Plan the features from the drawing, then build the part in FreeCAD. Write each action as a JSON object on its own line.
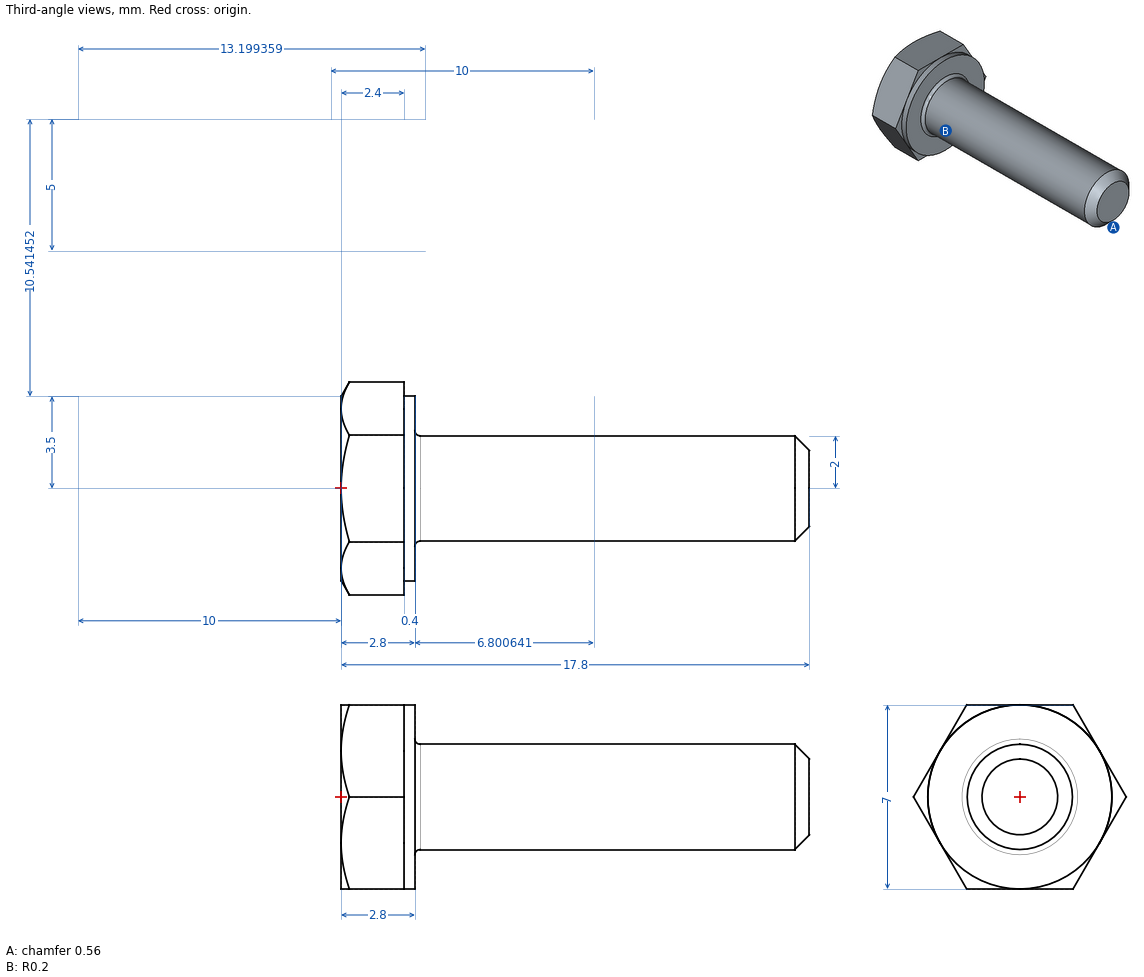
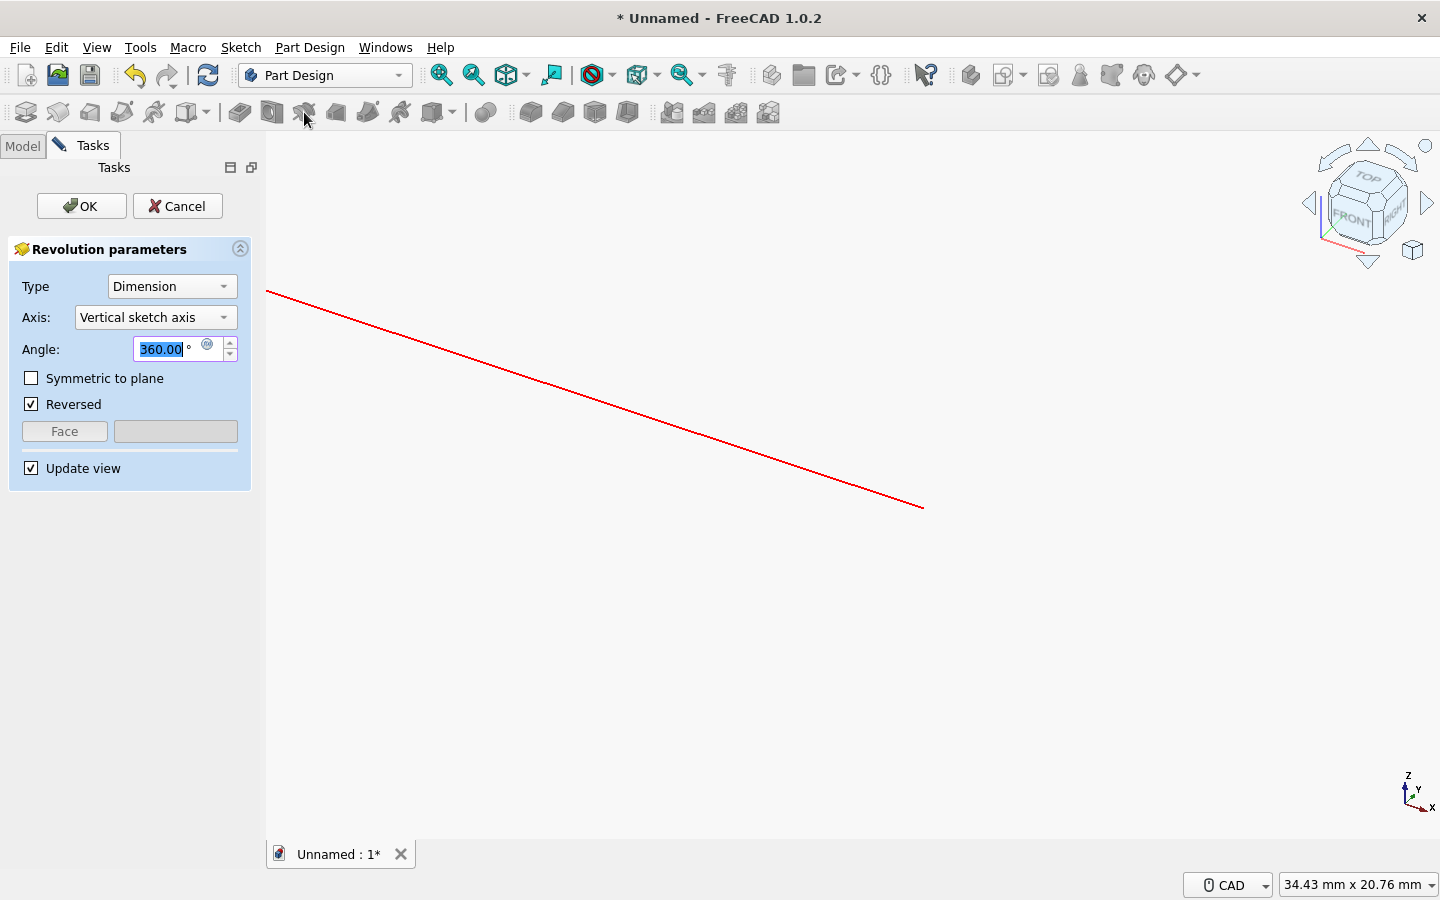
{"action": "left_click", "coordinate": [156, 318]}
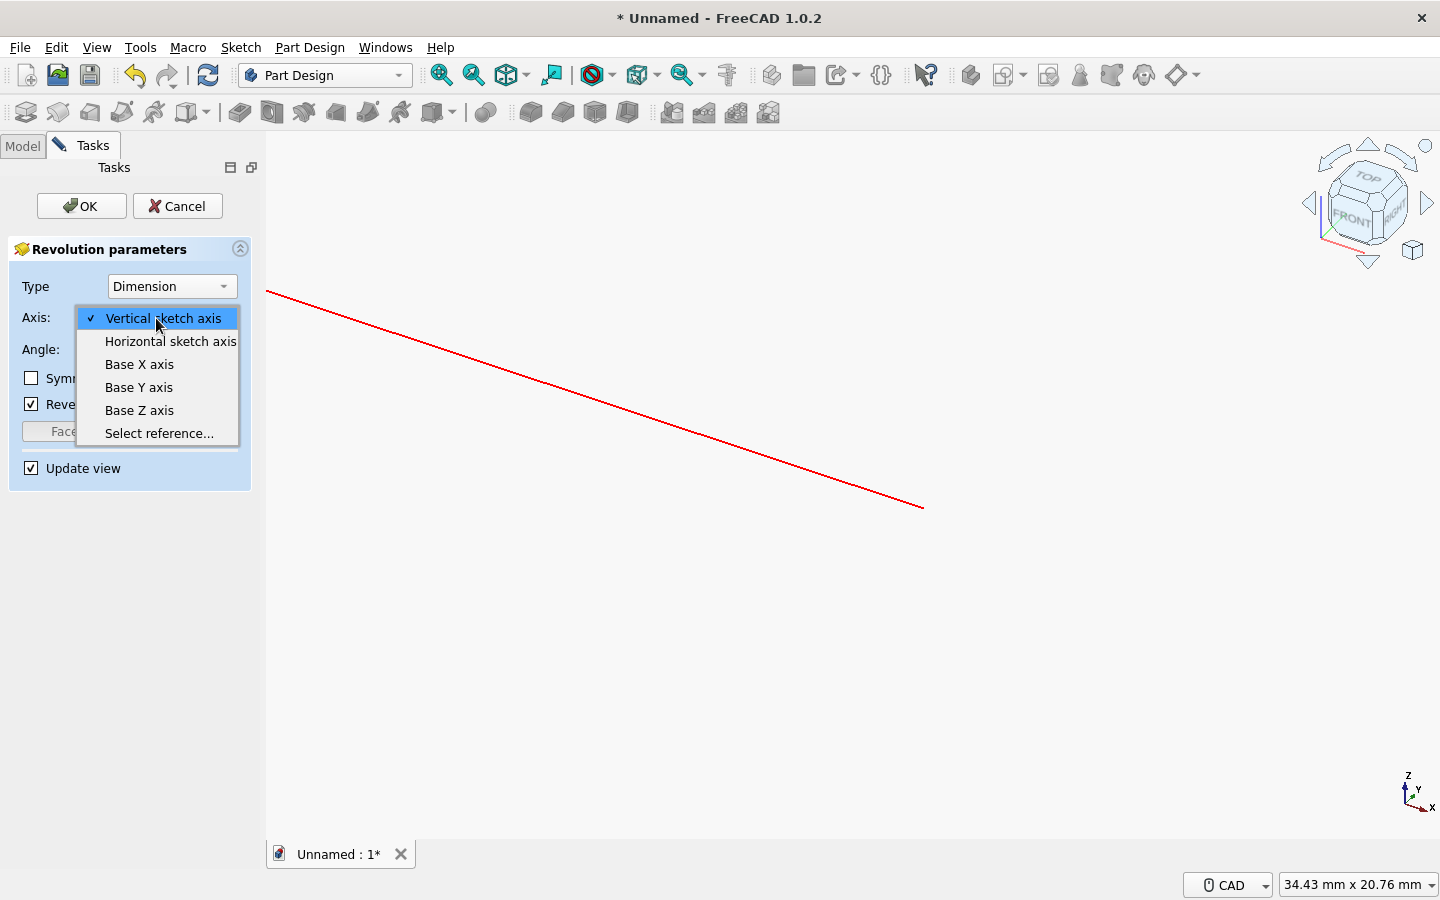
{"action": "left_click", "coordinate": [156, 342]}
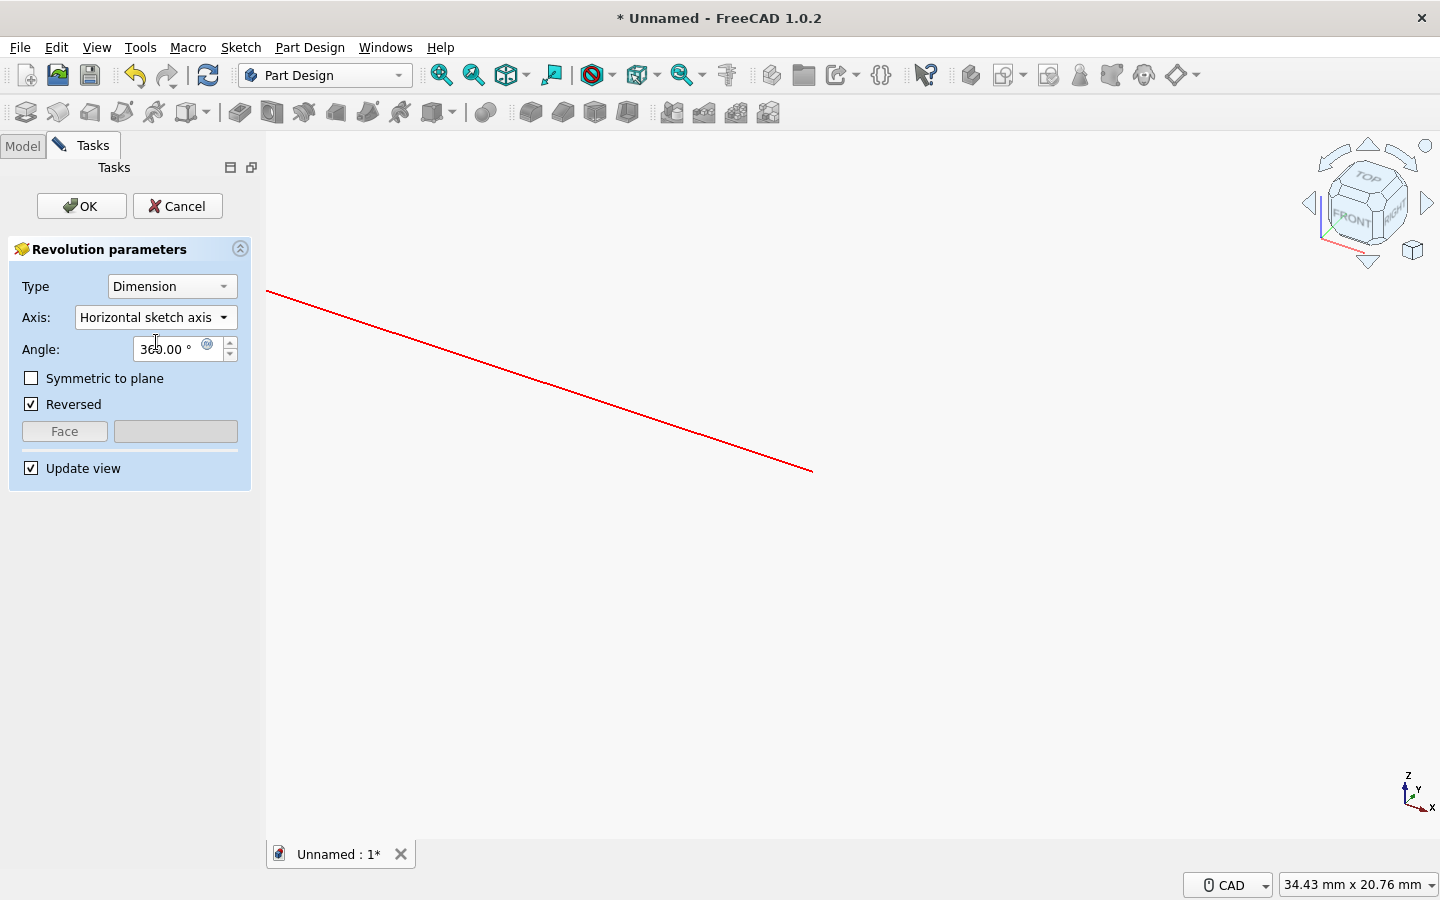
{"action": "left_click", "coordinate": [82, 206]}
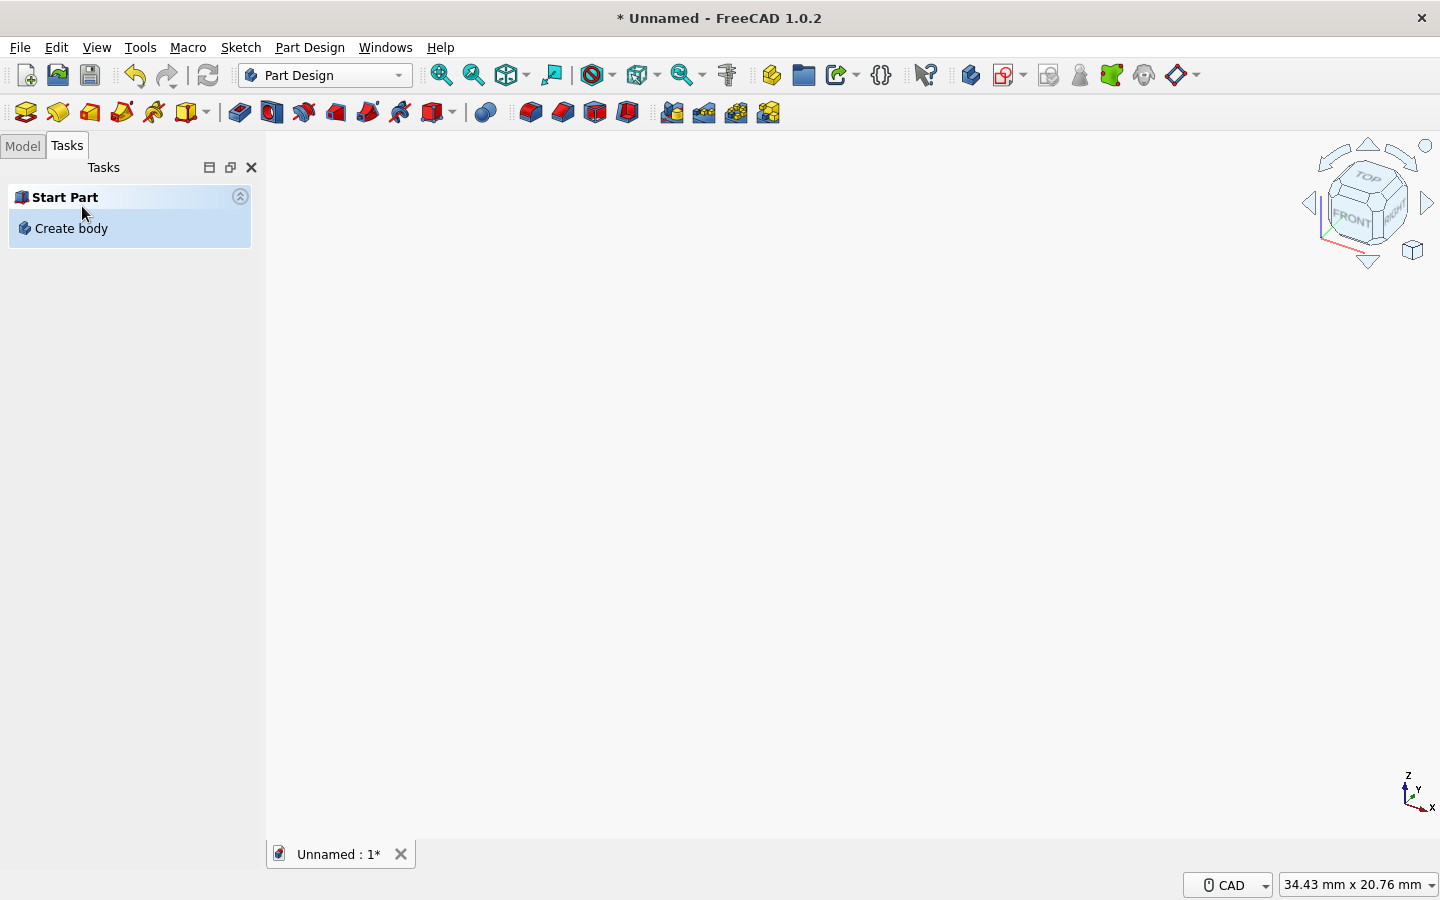
{"action": "key", "text": "v f"}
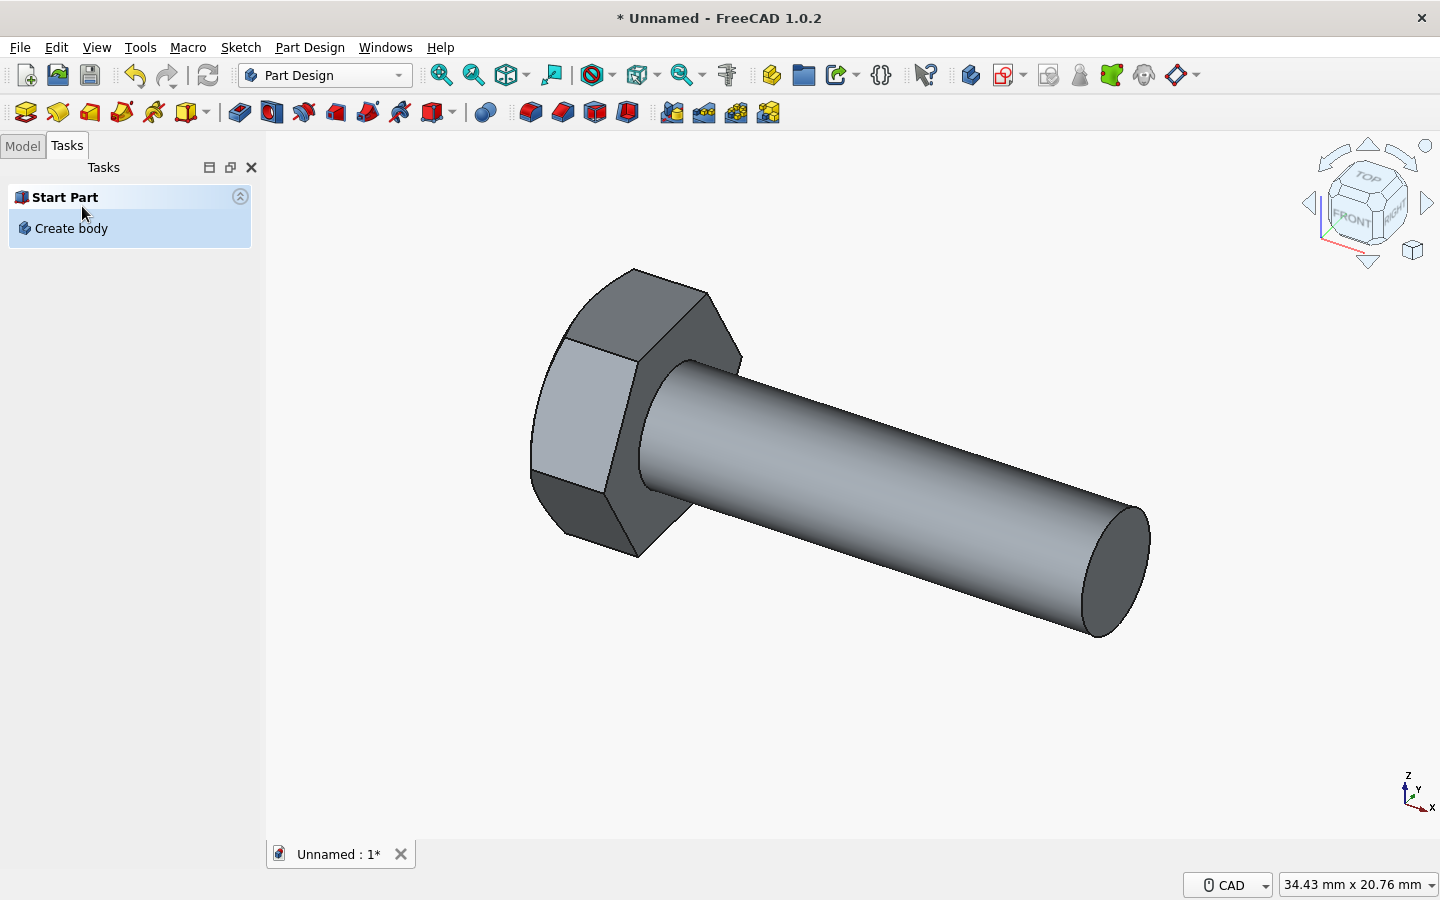
{"action": "left_click", "coordinate": [1004, 76]}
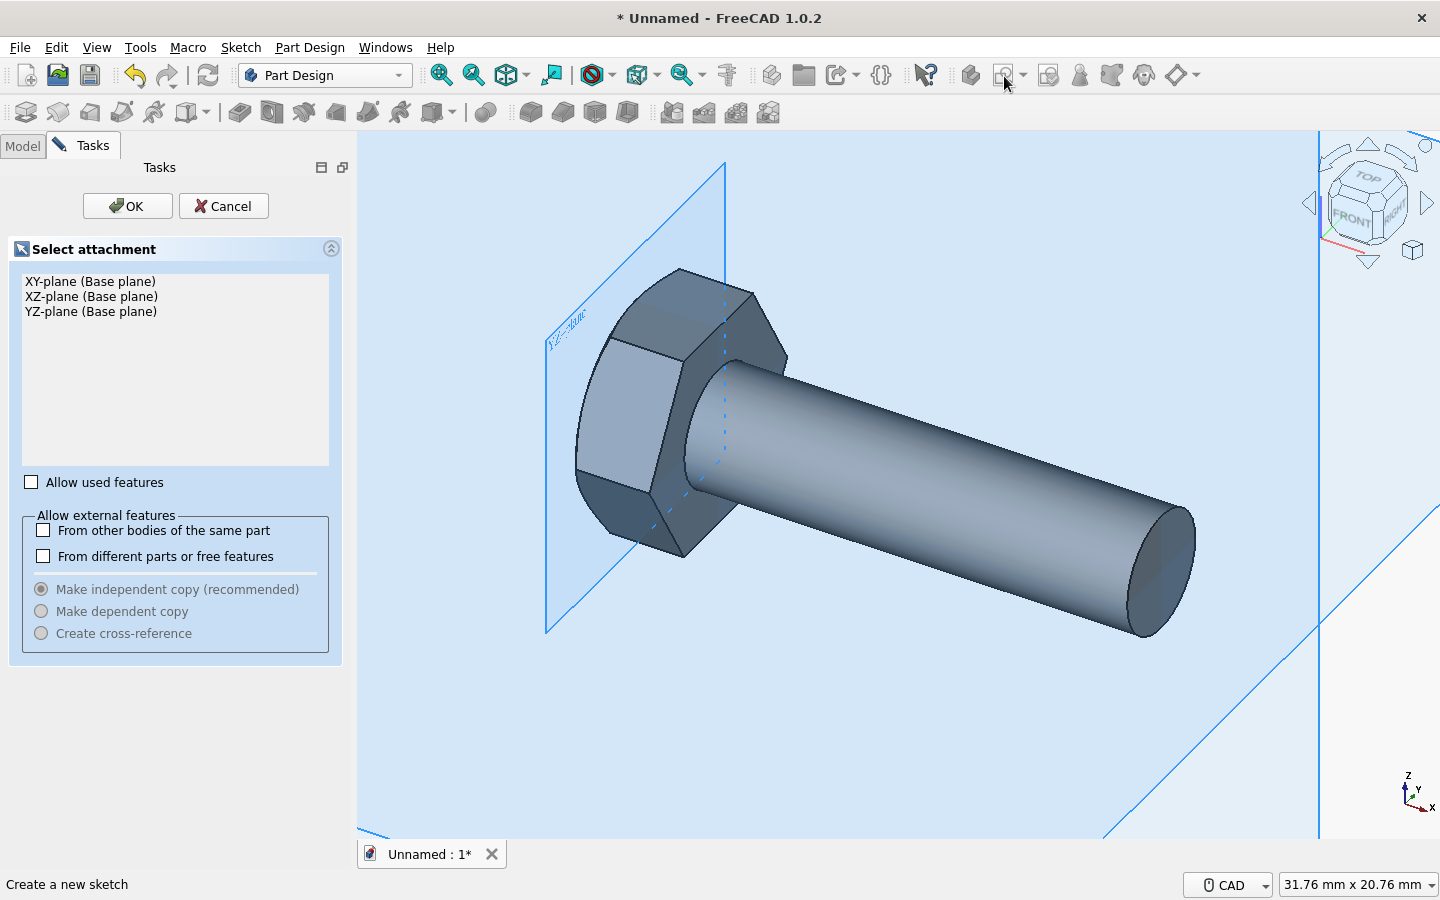
{"action": "left_click", "coordinate": [82, 282]}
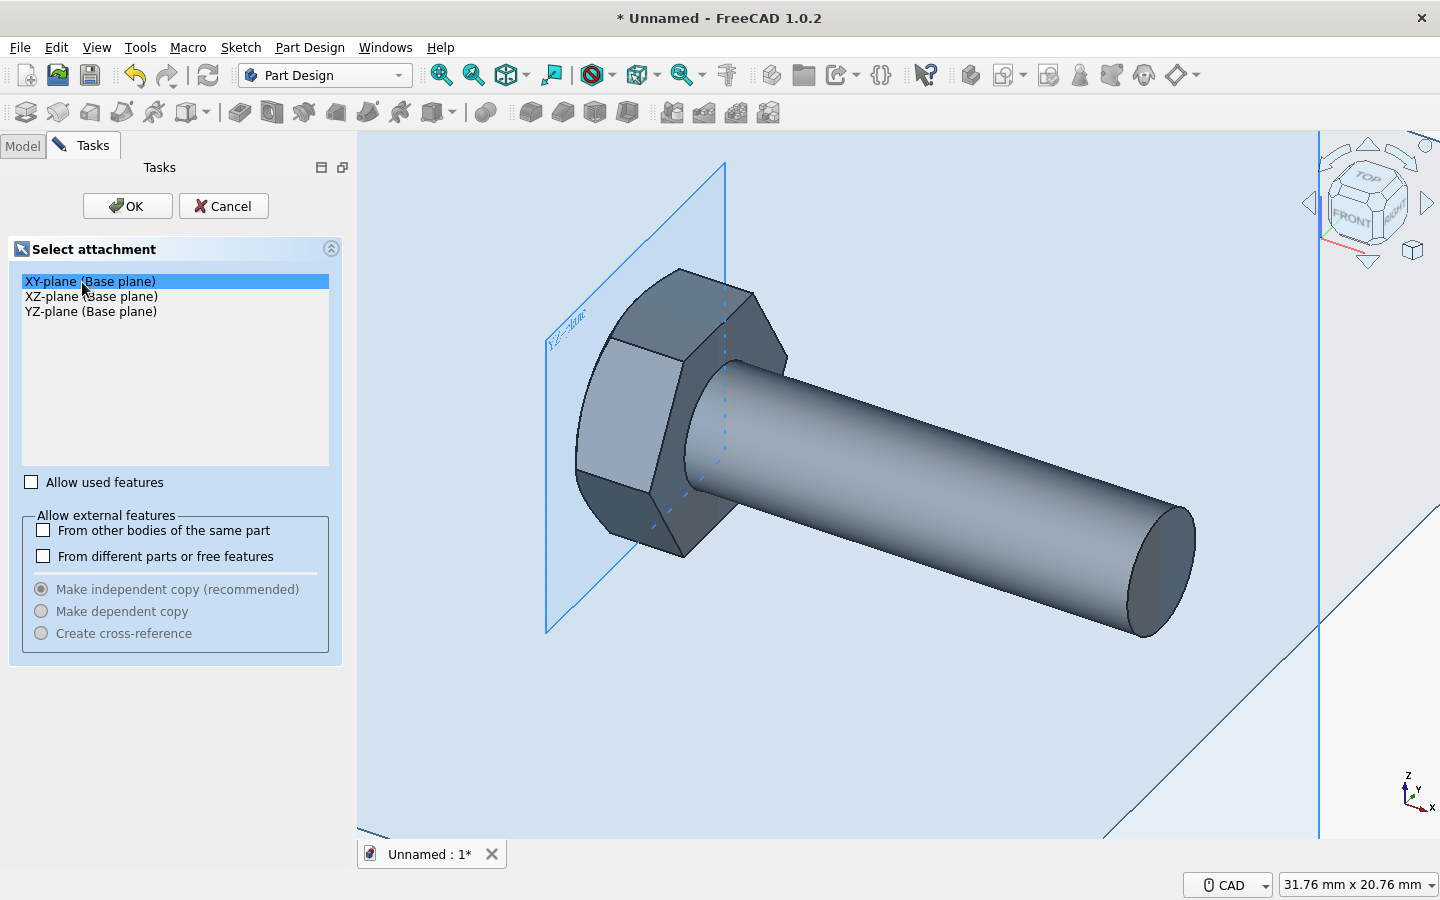
{"action": "left_click", "coordinate": [128, 206]}